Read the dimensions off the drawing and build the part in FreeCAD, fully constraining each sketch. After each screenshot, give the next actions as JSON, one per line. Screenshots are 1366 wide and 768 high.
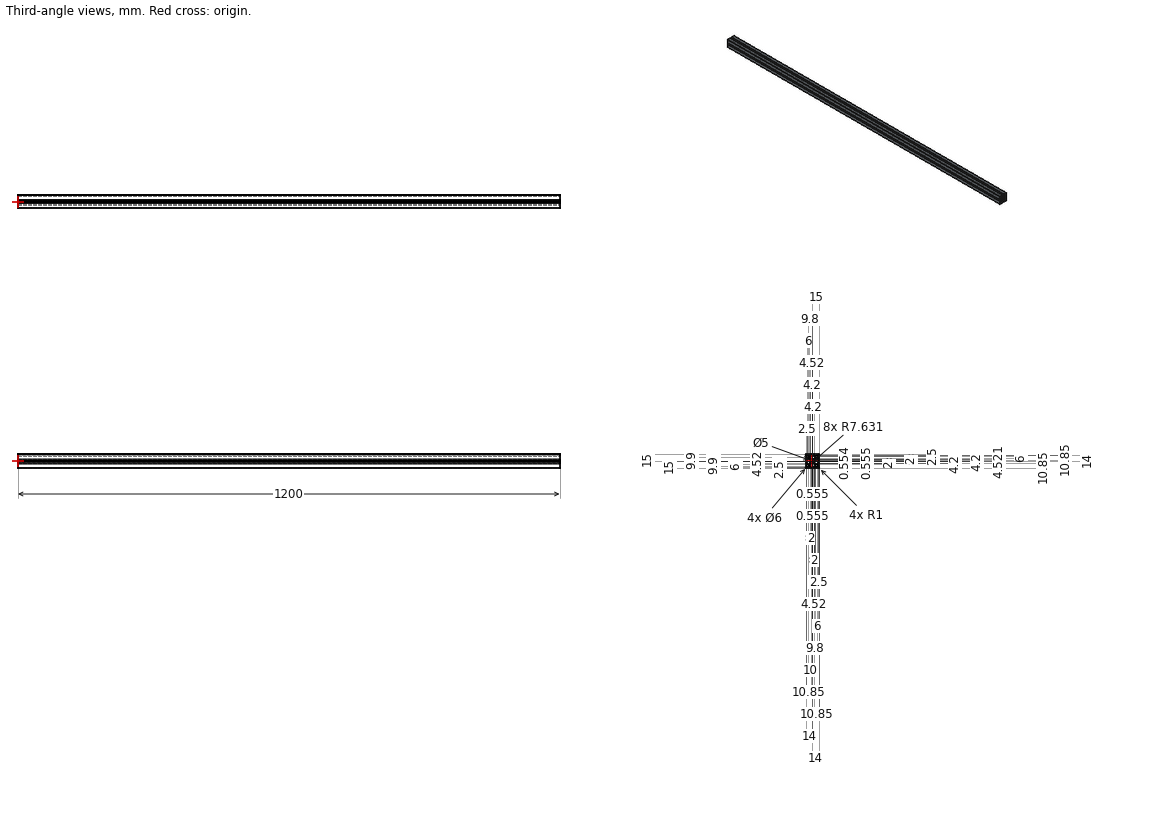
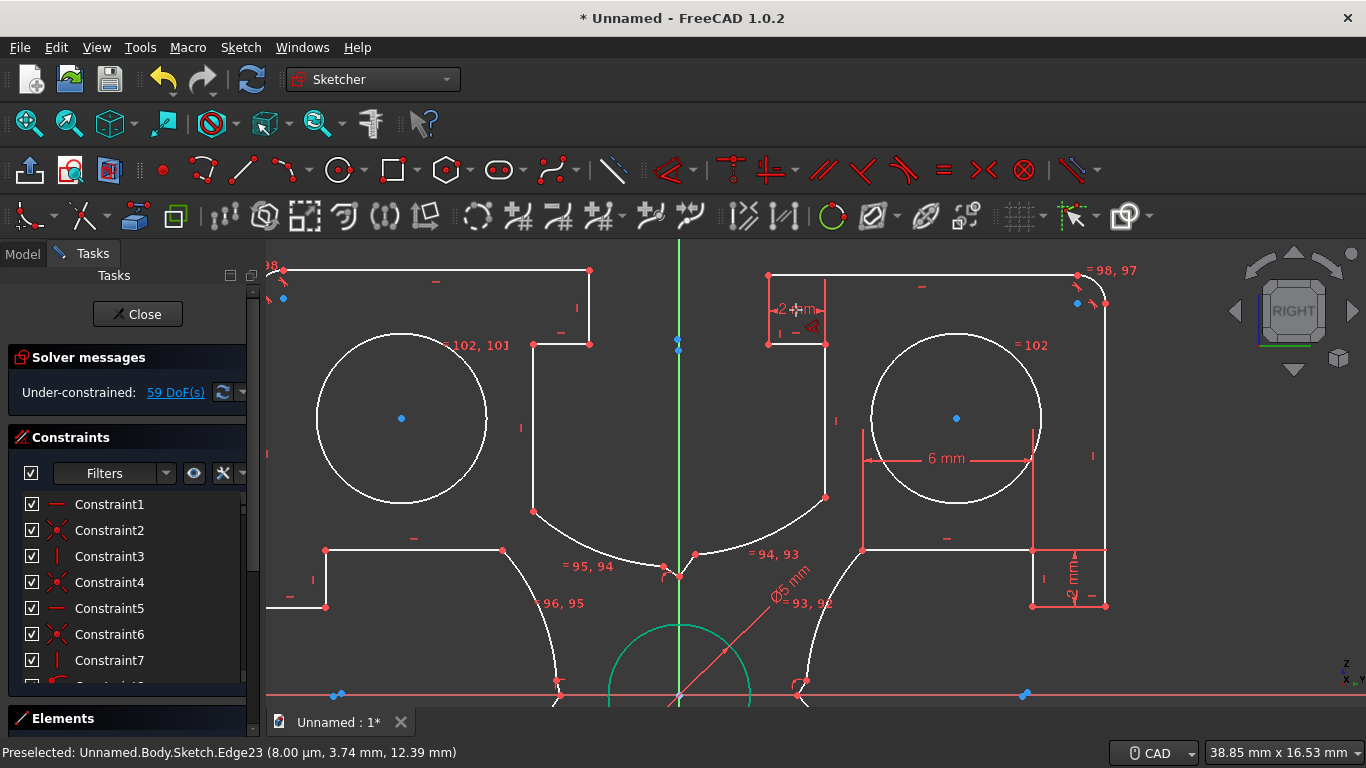
{"action": "left_click", "coordinate": [825, 390]}
{"action": "left_click", "coordinate": [859, 386]}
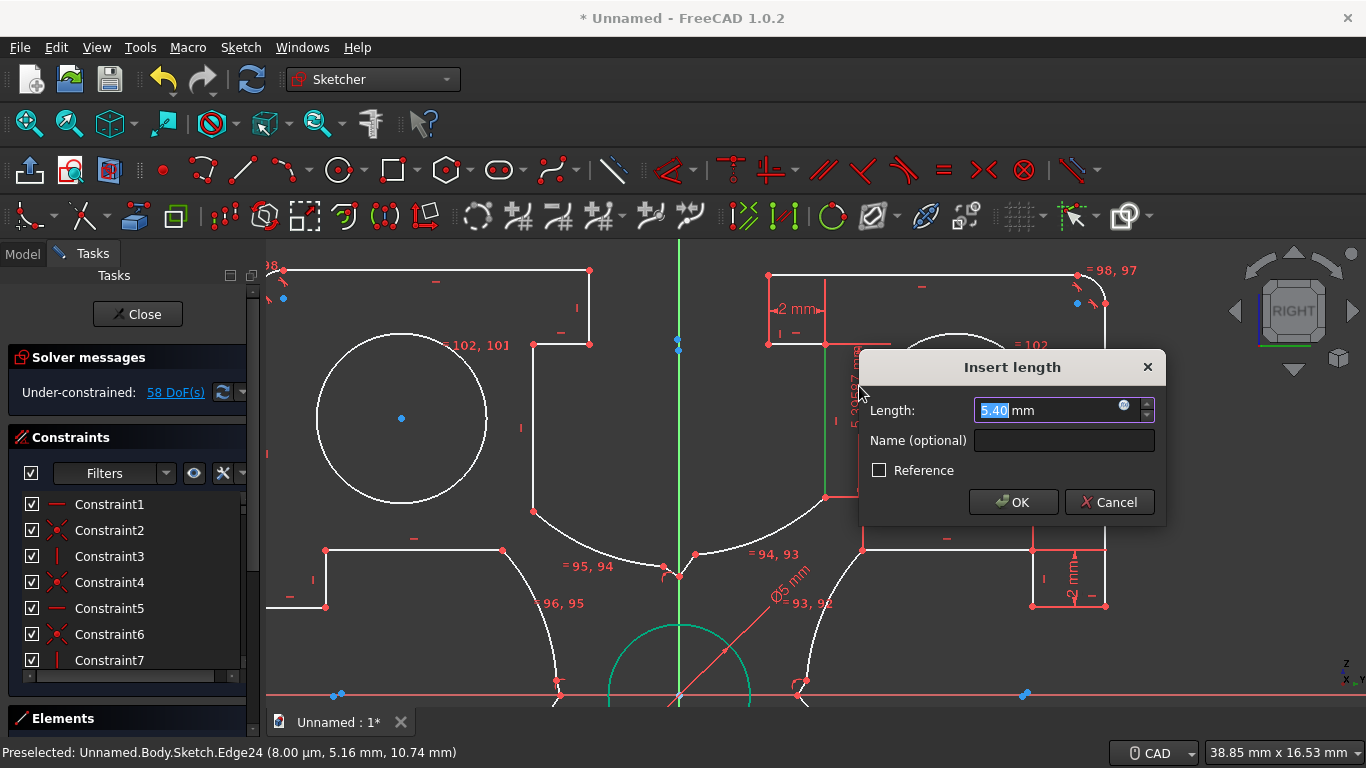
{"action": "type", "text": "6"}
{"action": "key", "text": "Return"}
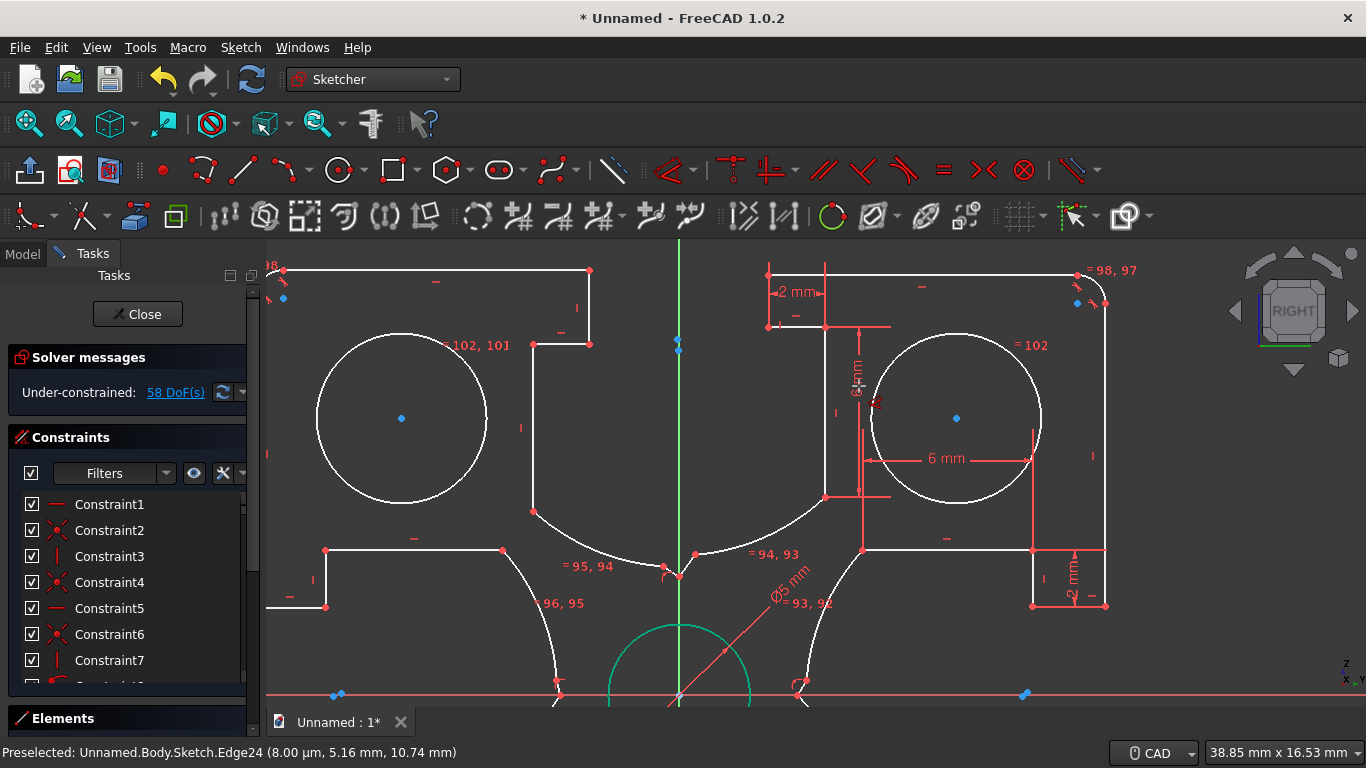
{"action": "left_click", "coordinate": [533, 461]}
{"action": "left_click", "coordinate": [499, 428]}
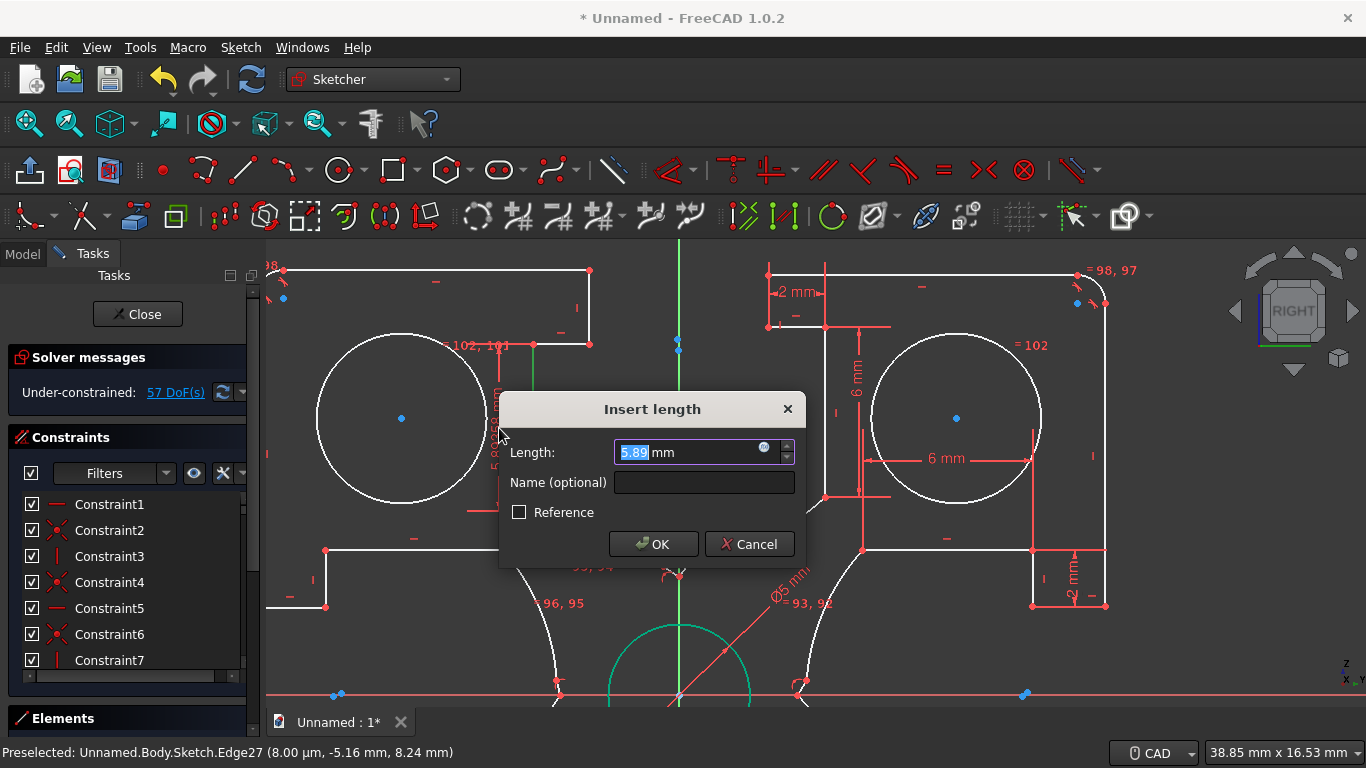
{"action": "type", "text": "6"}
{"action": "key", "text": "Return"}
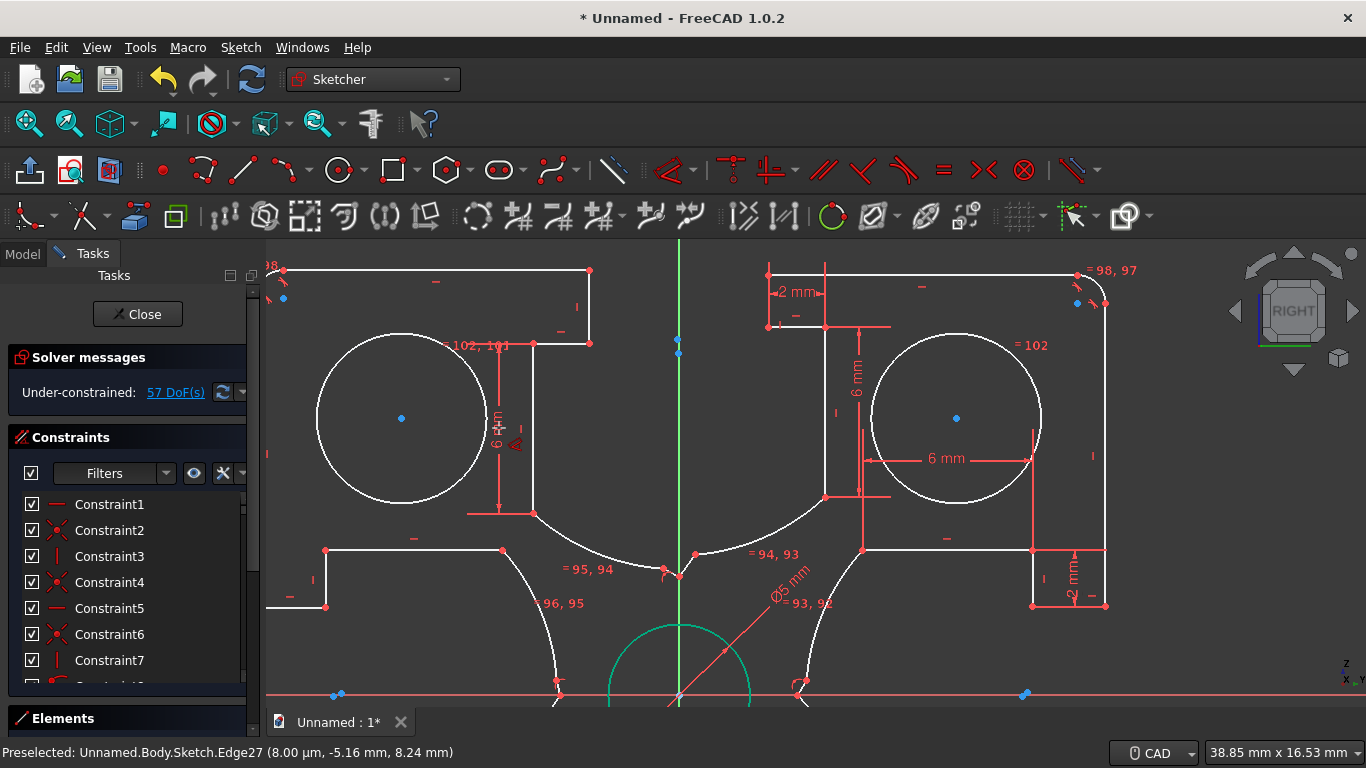
{"action": "left_click", "coordinate": [550, 344]}
{"action": "left_click", "coordinate": [561, 310]}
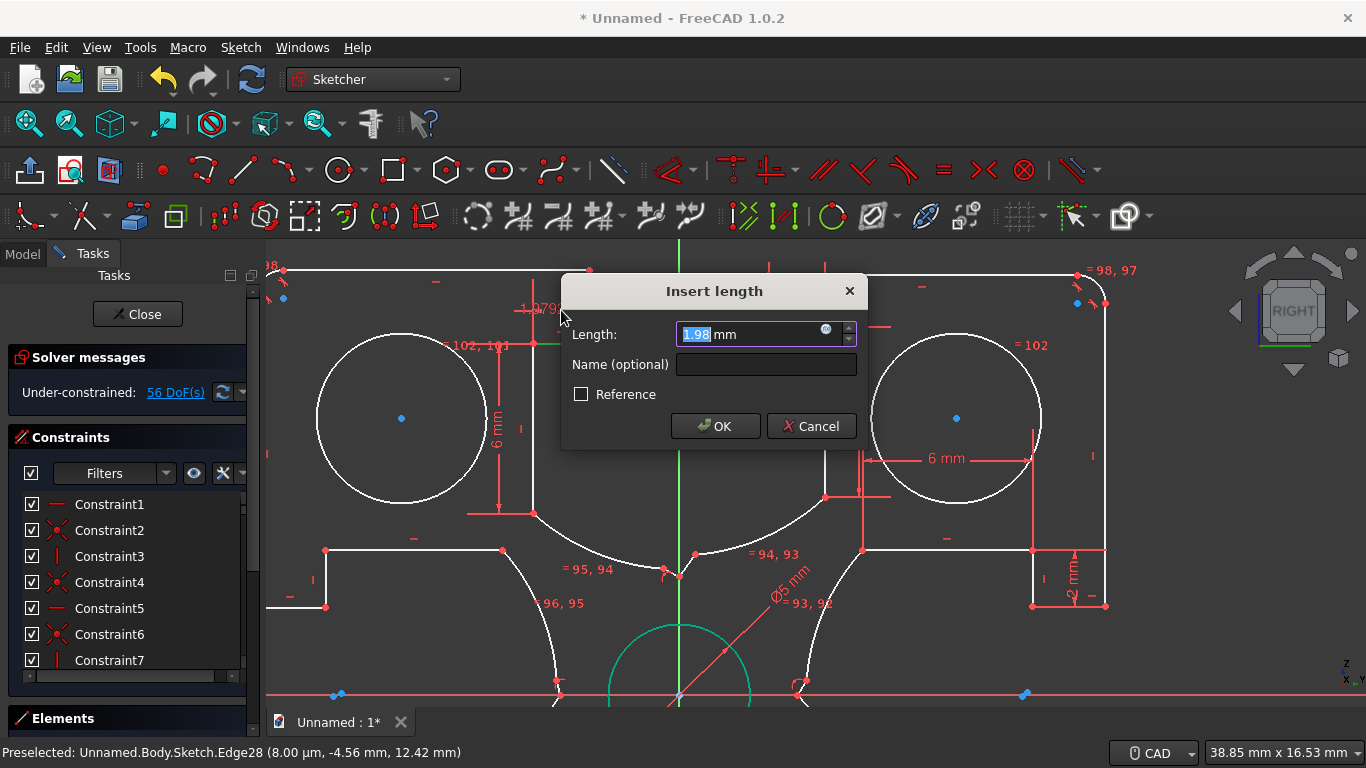
{"action": "type", "text": "2"}
{"action": "key", "text": "Return"}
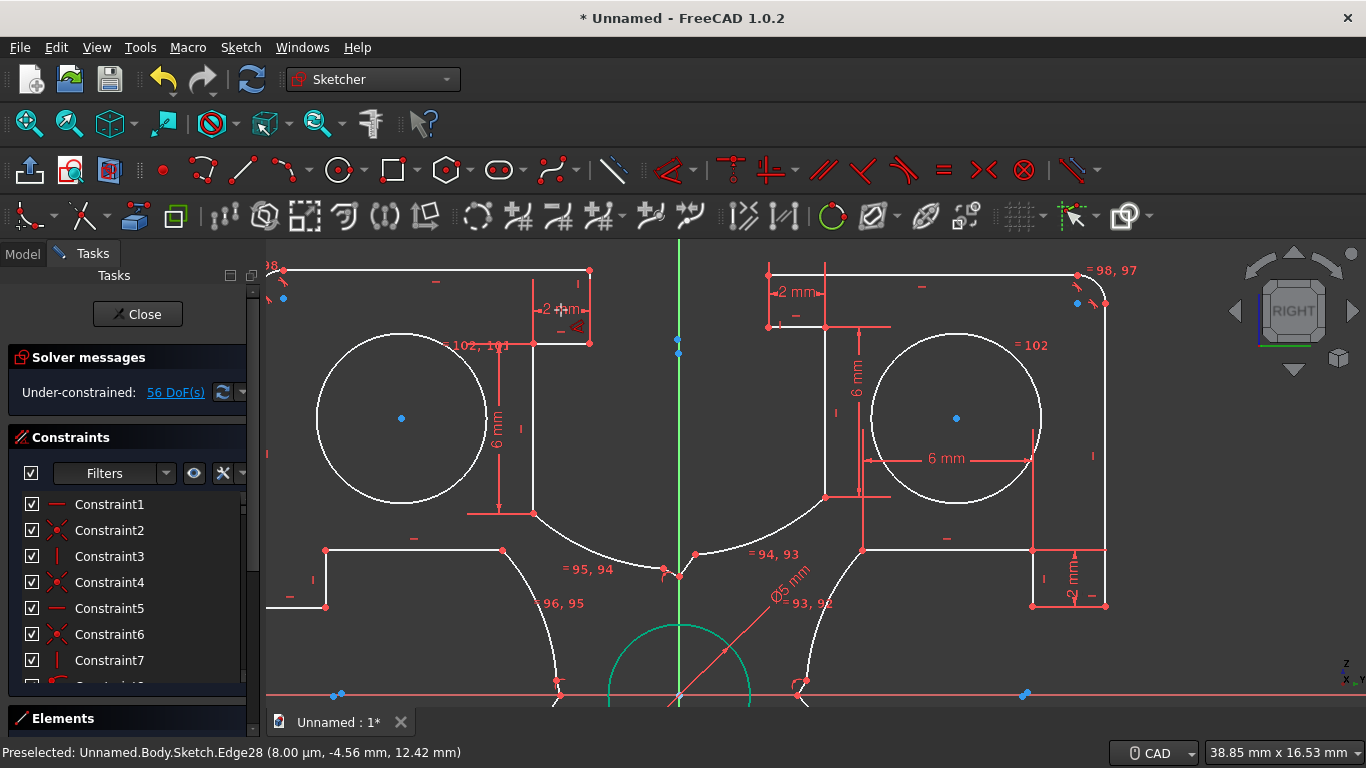
{"action": "left_click", "coordinate": [326, 591]}
{"action": "left_click", "coordinate": [360, 579]}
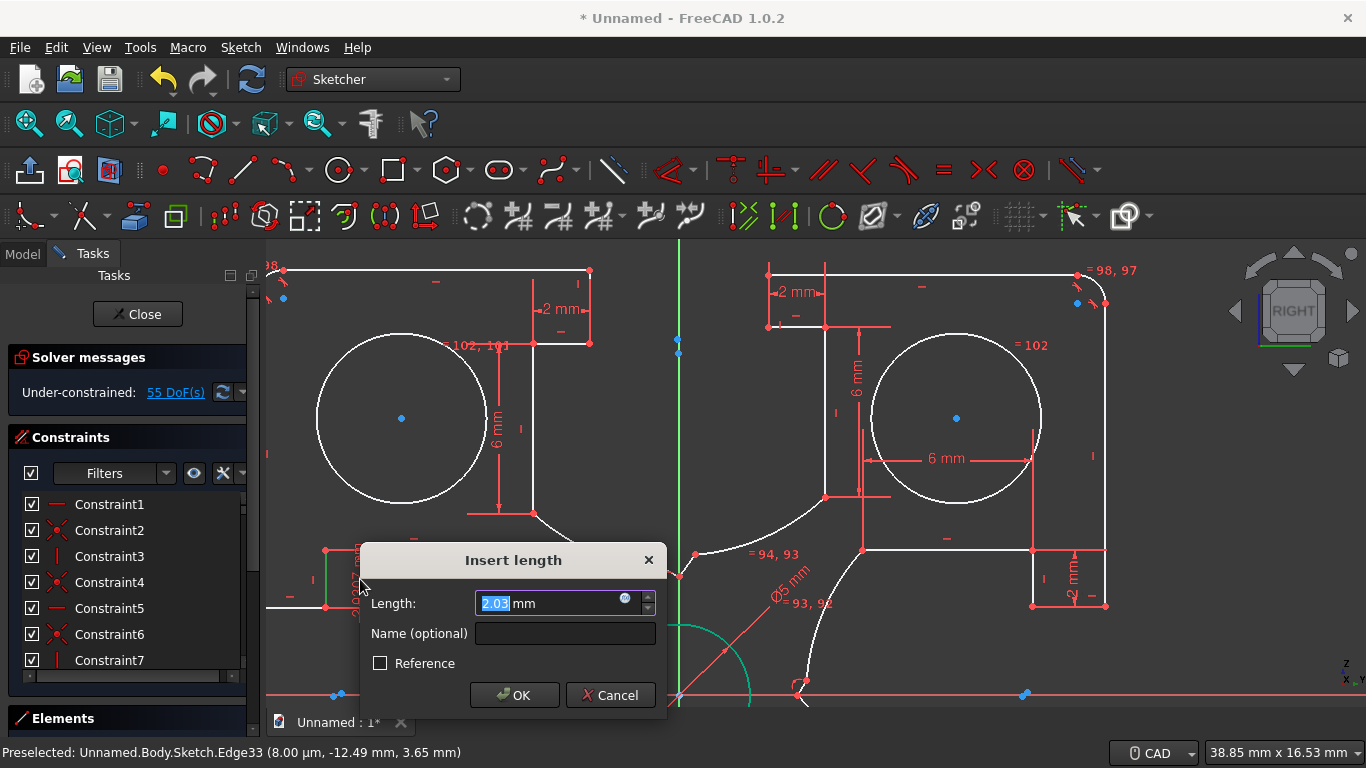
{"action": "type", "text": "2"}
{"action": "key", "text": "Return"}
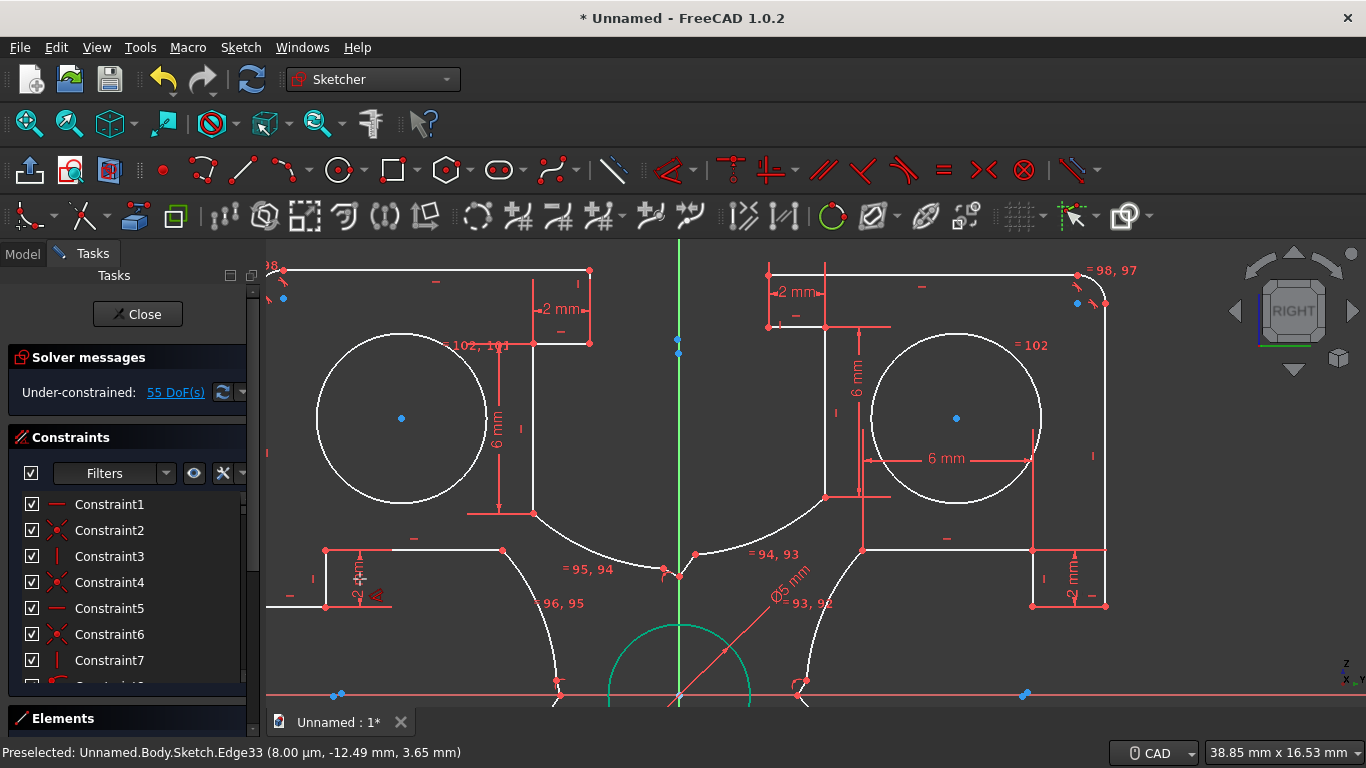
{"action": "left_click", "coordinate": [379, 550]}
{"action": "left_click", "coordinate": [414, 516]}